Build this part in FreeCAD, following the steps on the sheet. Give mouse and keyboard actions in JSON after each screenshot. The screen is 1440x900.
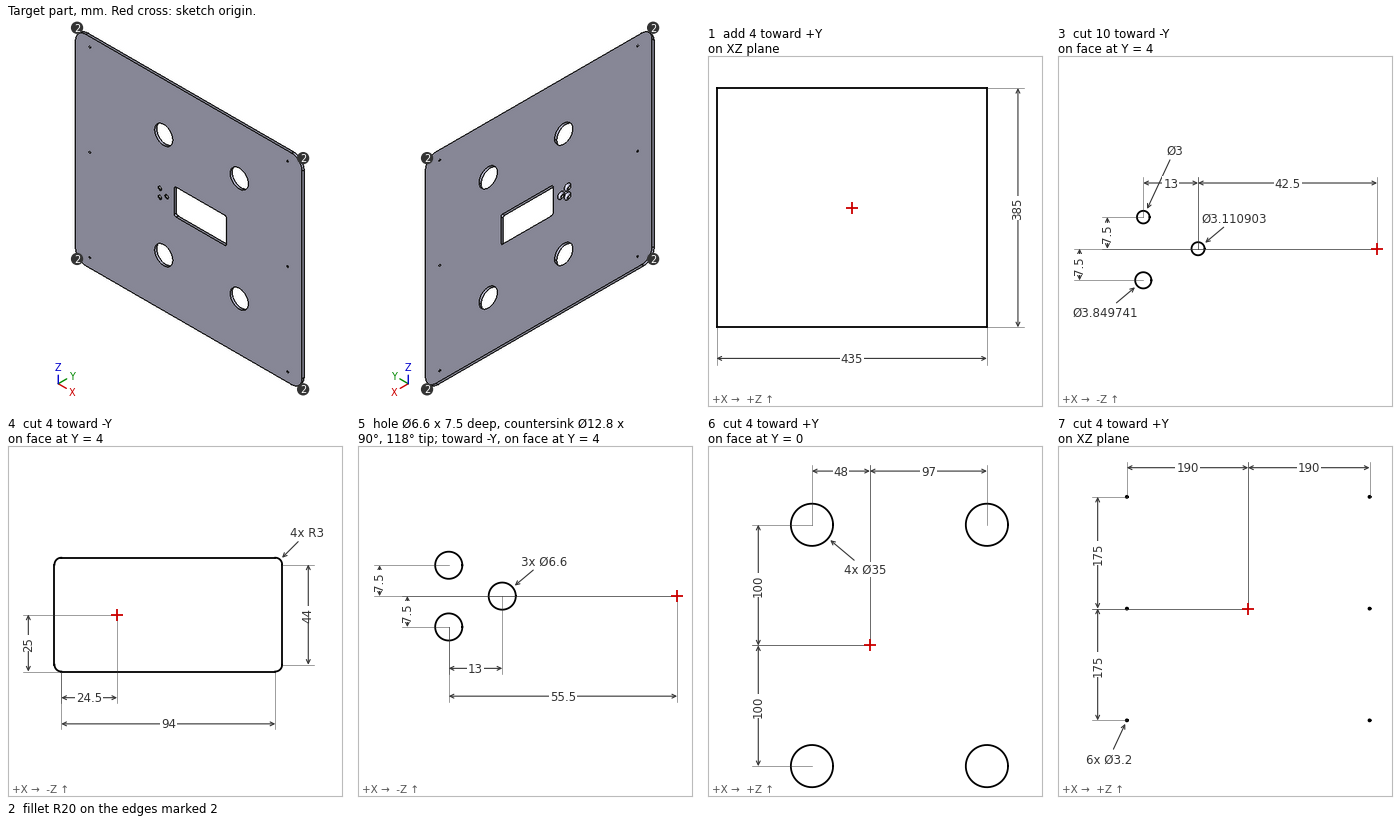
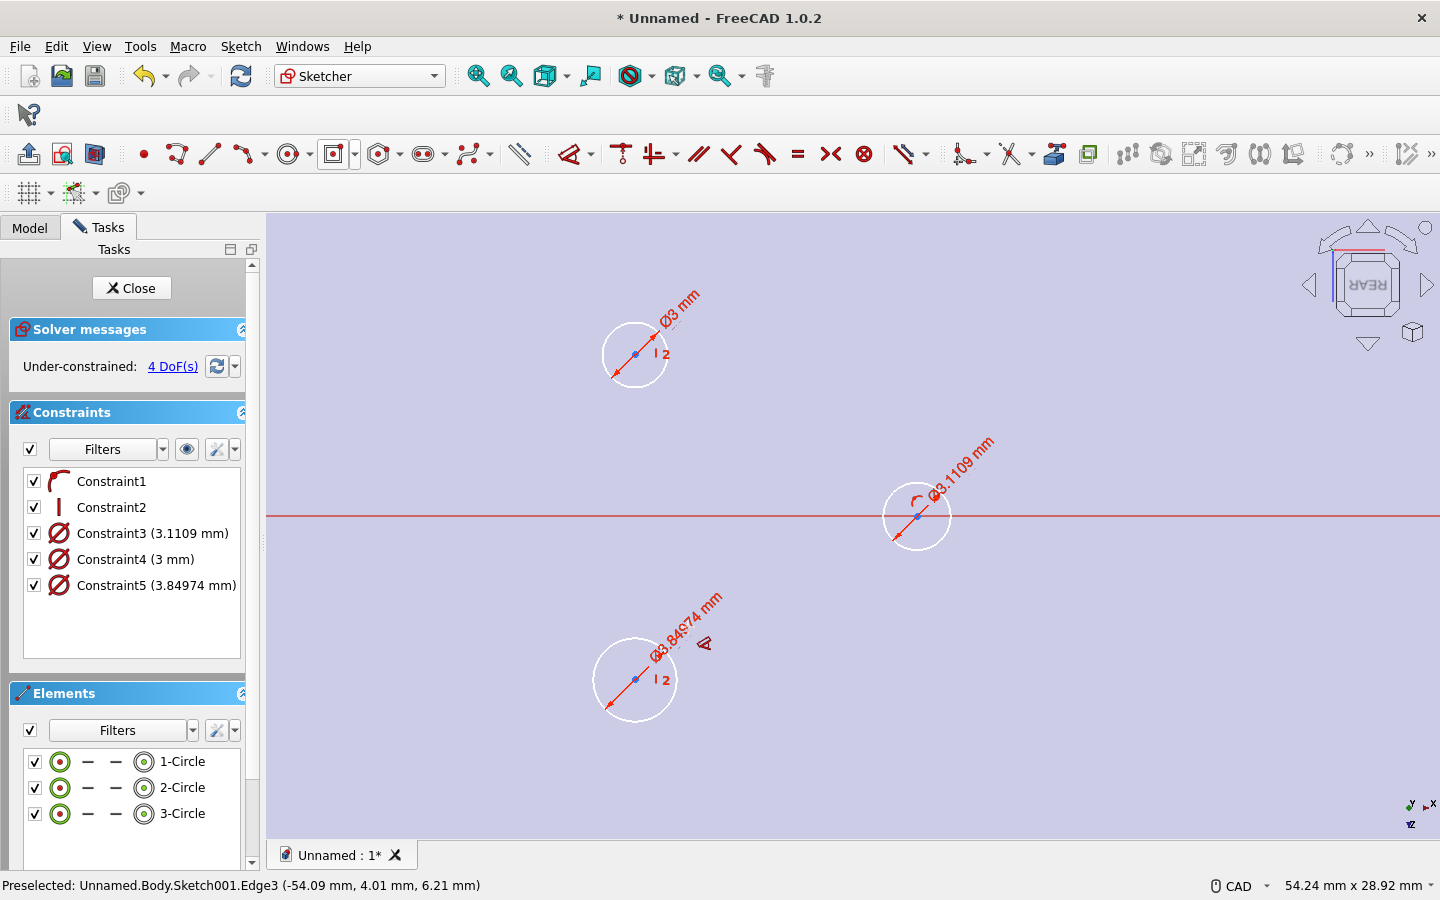
{"action": "left_click", "coordinate": [635, 355]}
{"action": "left_click", "coordinate": [601, 436]}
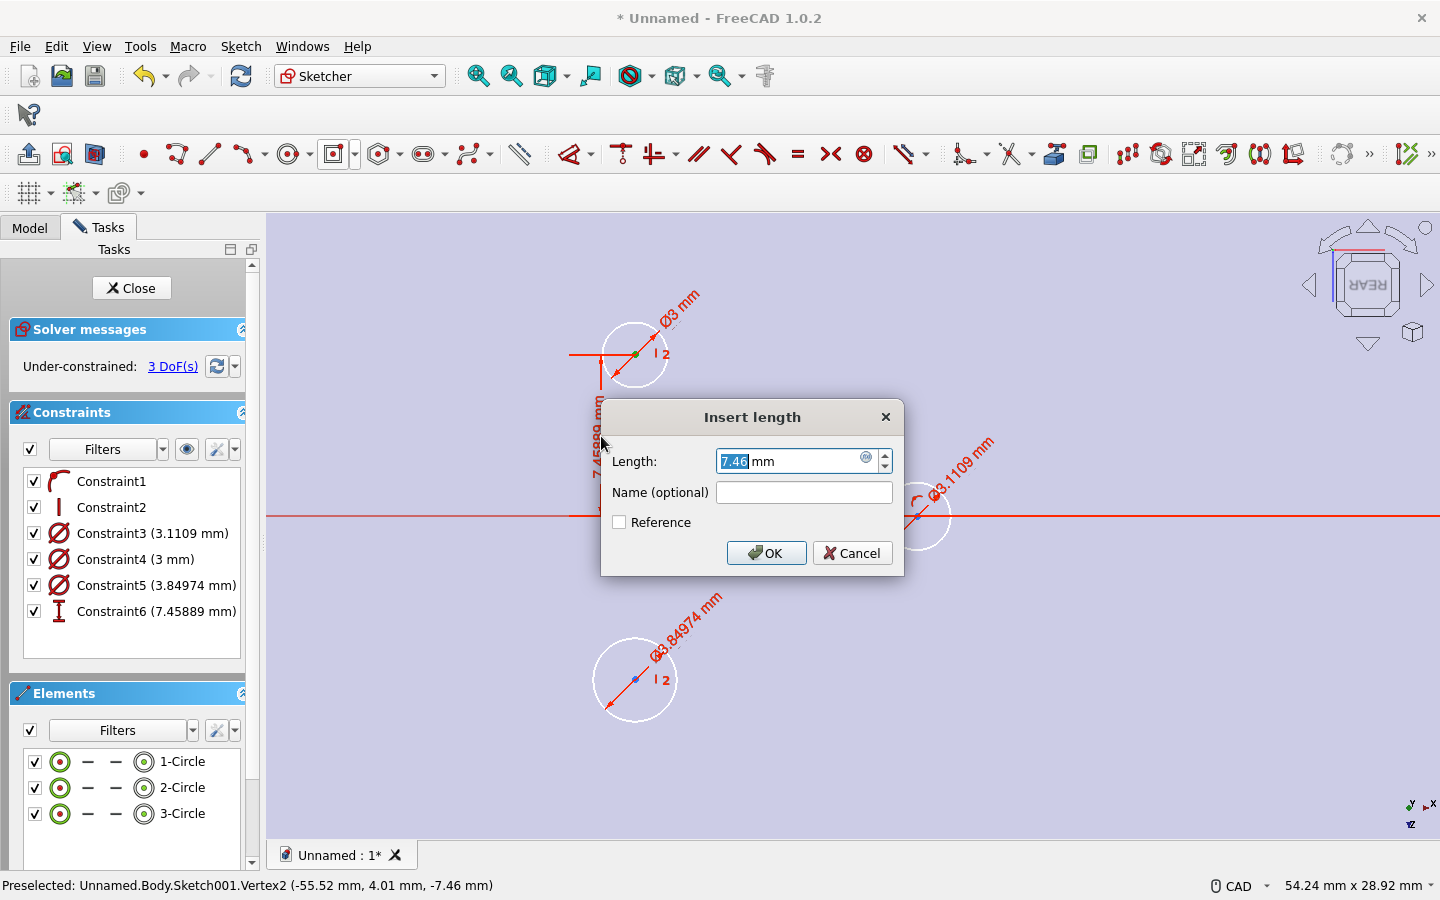
{"action": "type", "text": "7.5"}
{"action": "key", "text": "Return"}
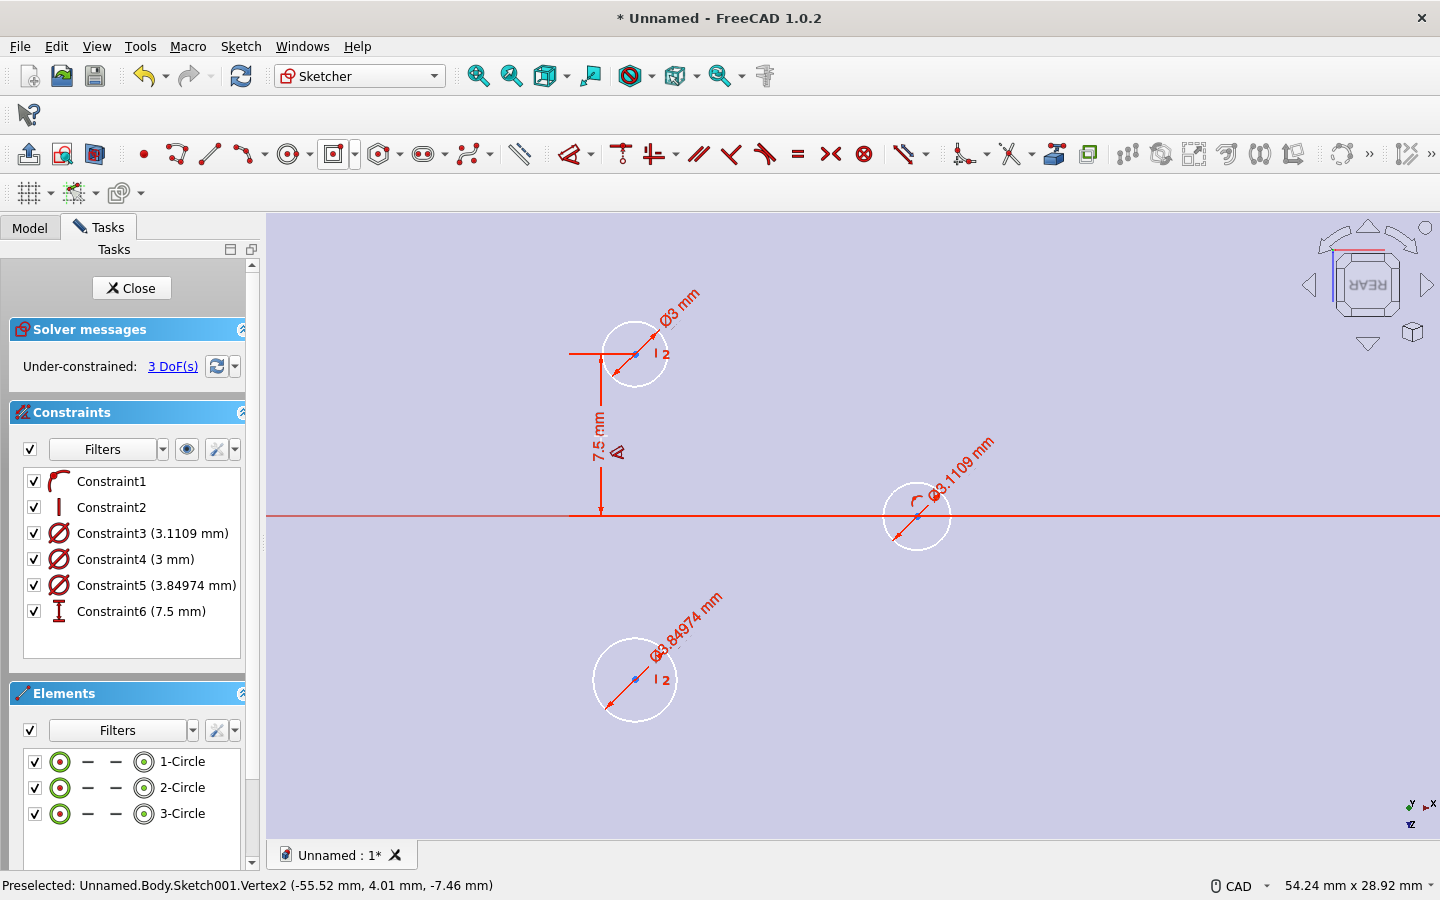
{"action": "left_click", "coordinate": [635, 680]}
{"action": "left_click", "coordinate": [601, 598]}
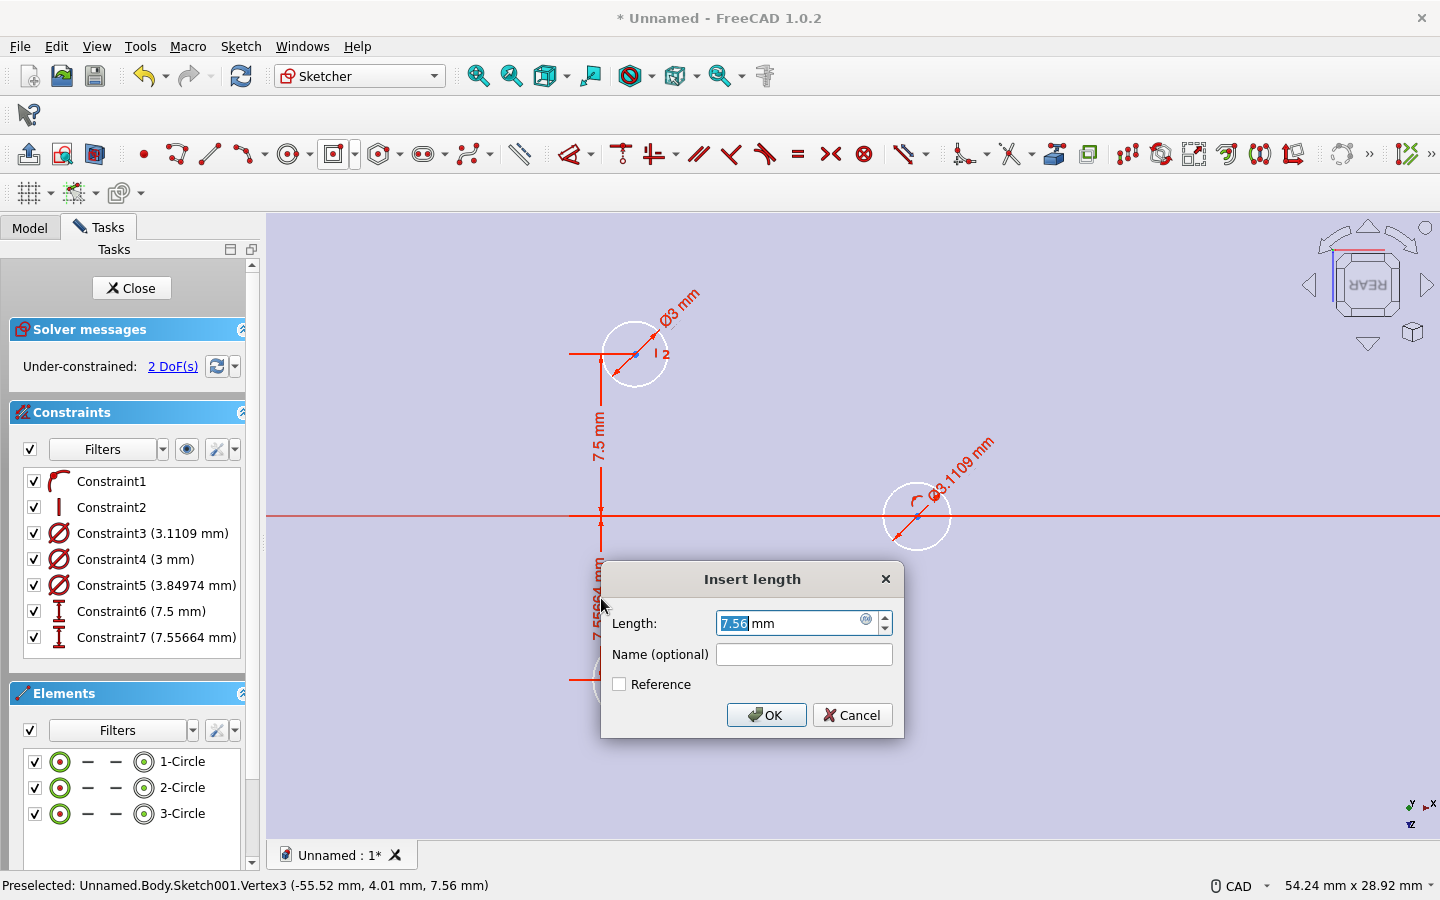
{"action": "type", "text": "7.5"}
{"action": "key", "text": "Return"}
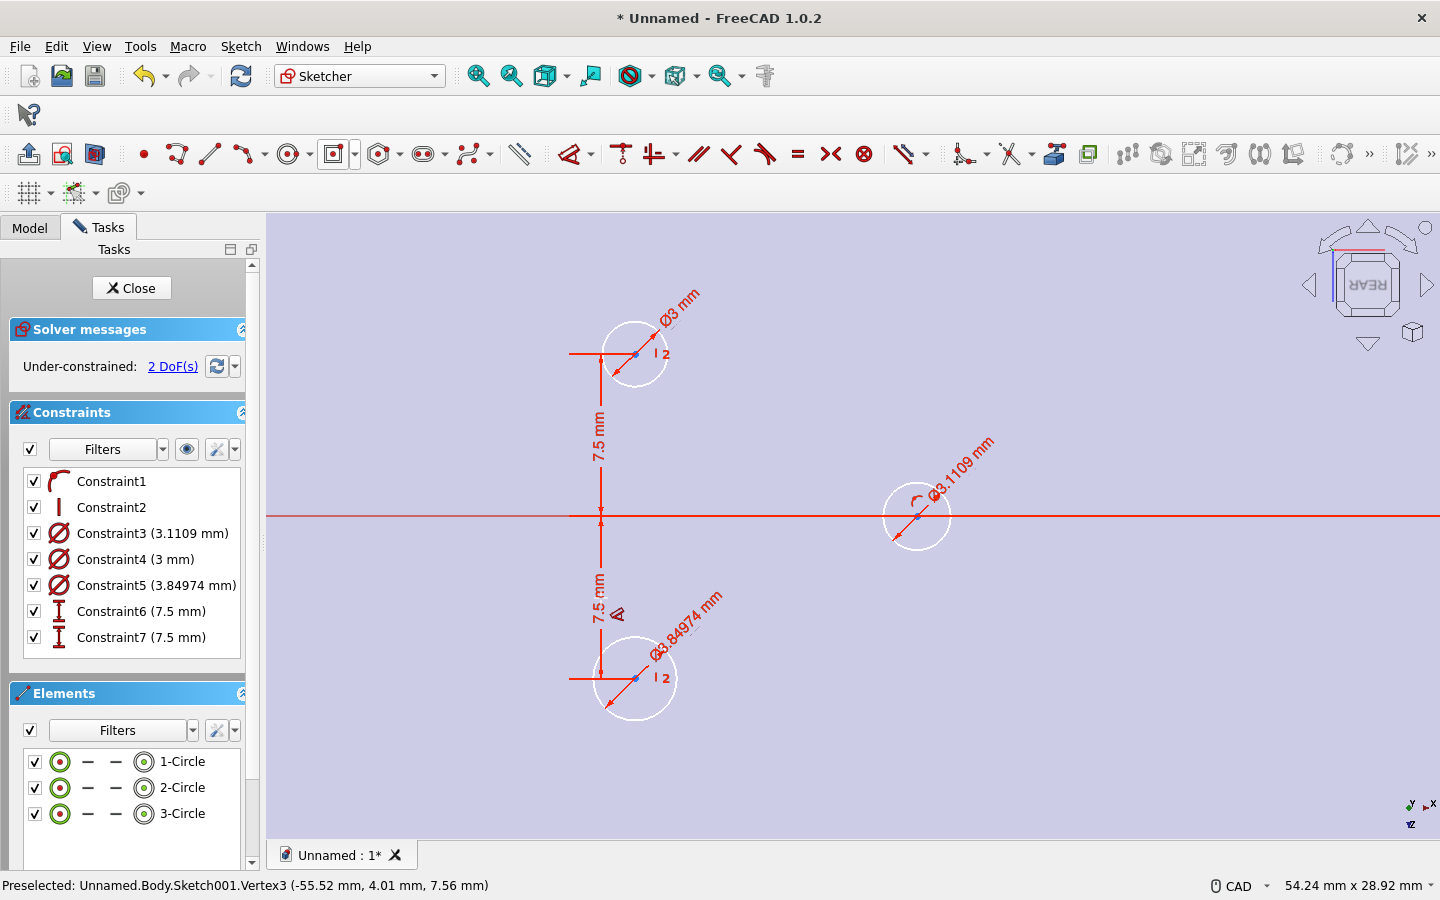
{"action": "left_click", "coordinate": [917, 516]}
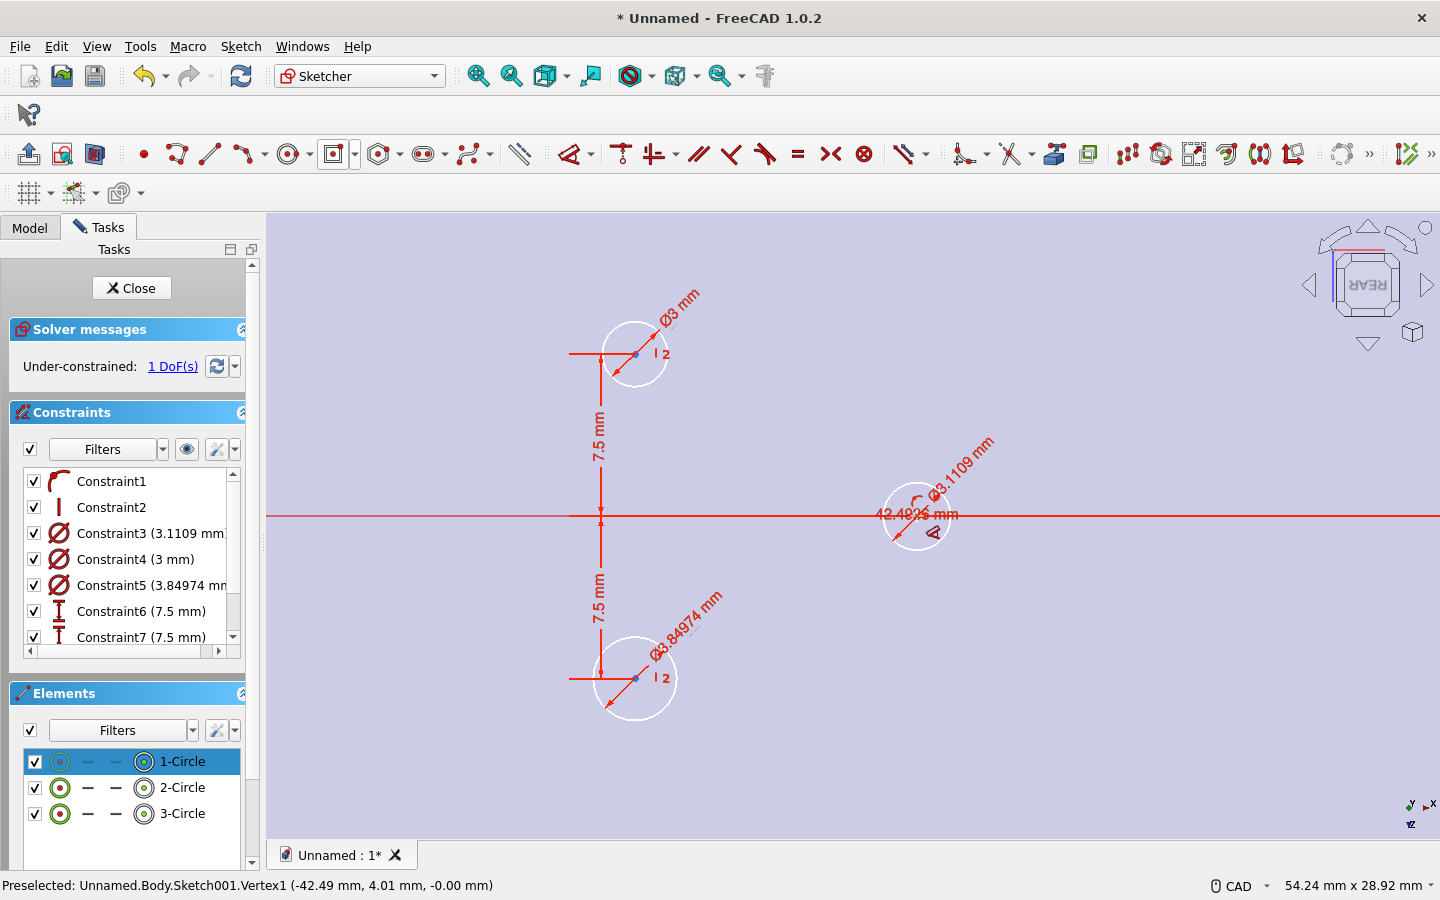
{"action": "left_click", "coordinate": [635, 354]}
{"action": "left_click", "coordinate": [776, 320]}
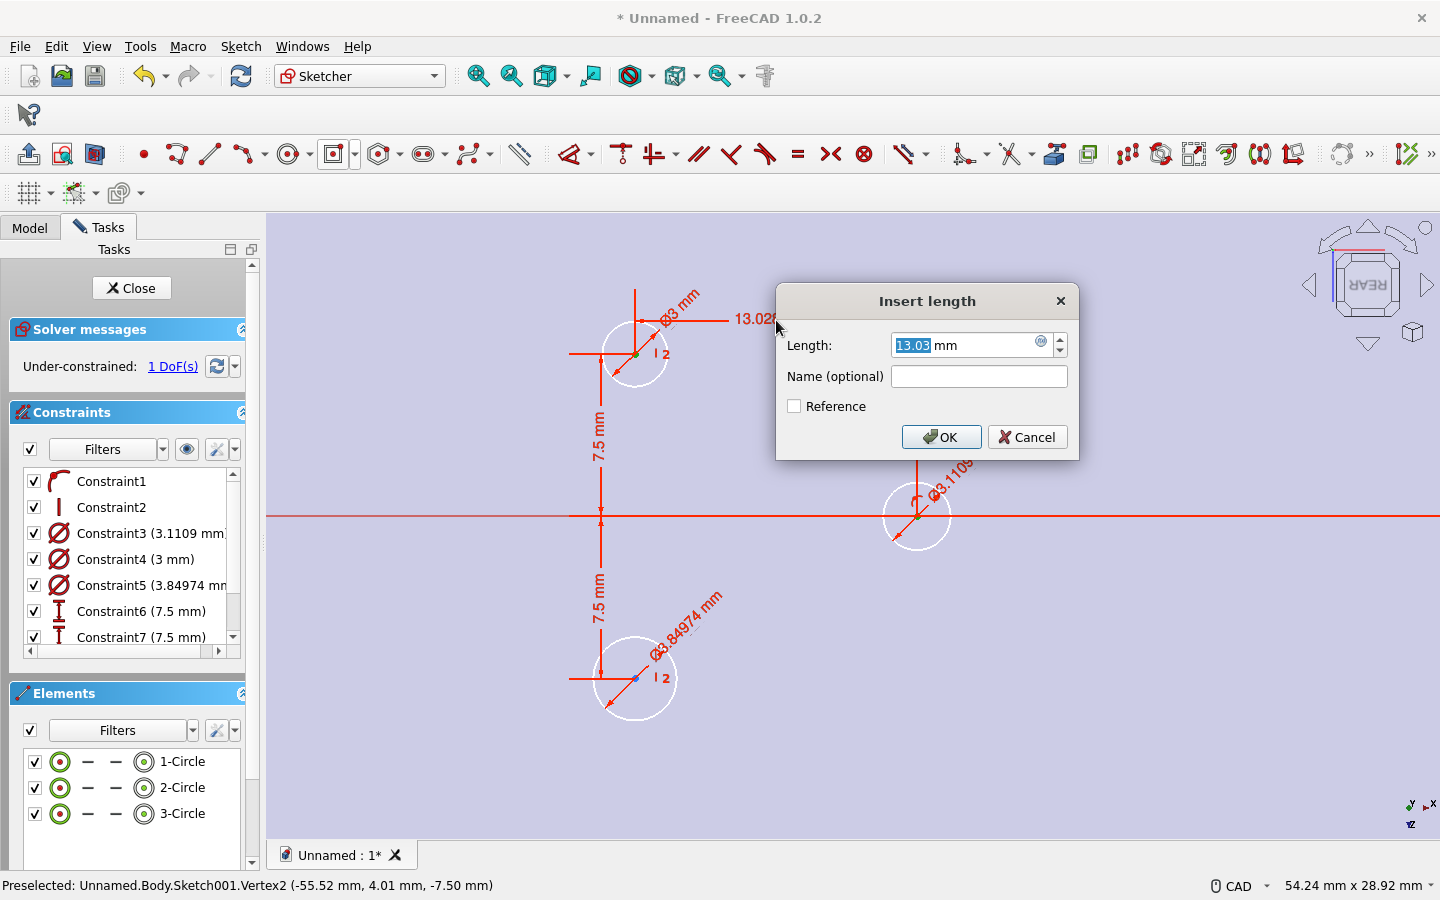
{"action": "type", "text": "13"}
{"action": "key", "text": "Return"}